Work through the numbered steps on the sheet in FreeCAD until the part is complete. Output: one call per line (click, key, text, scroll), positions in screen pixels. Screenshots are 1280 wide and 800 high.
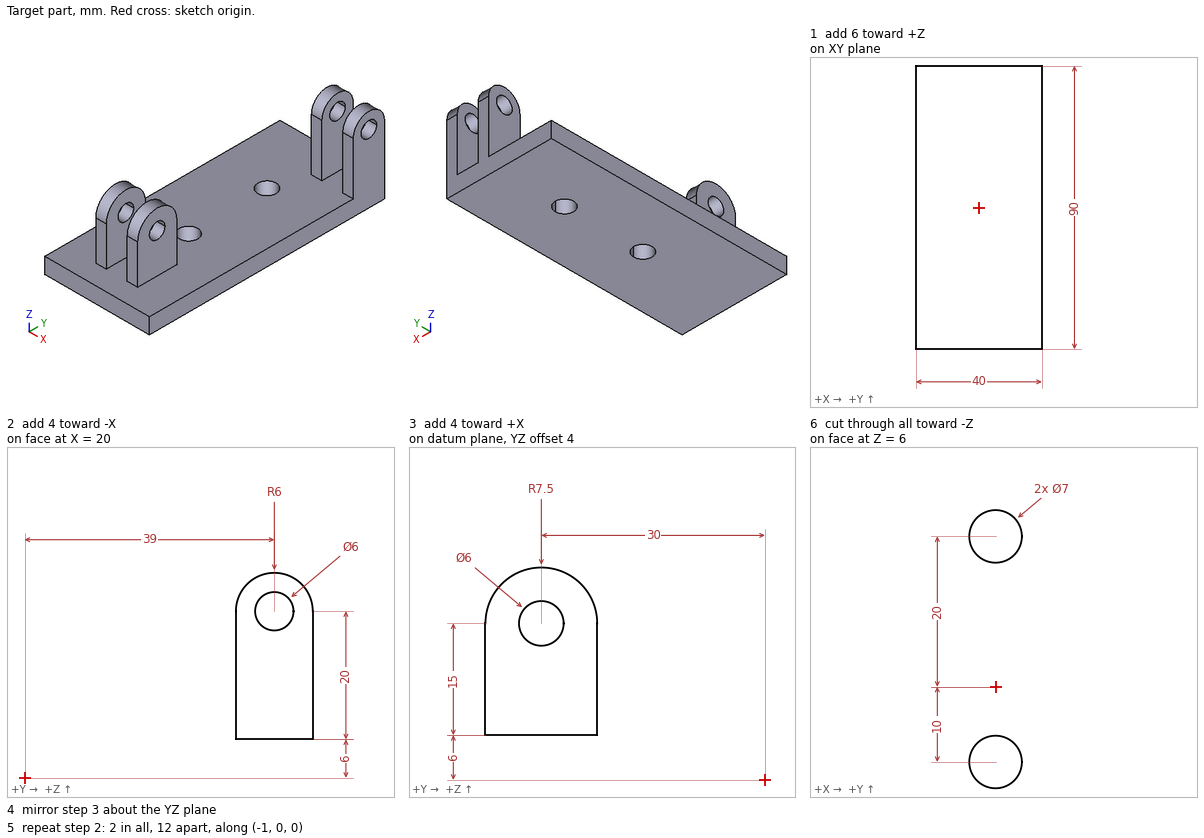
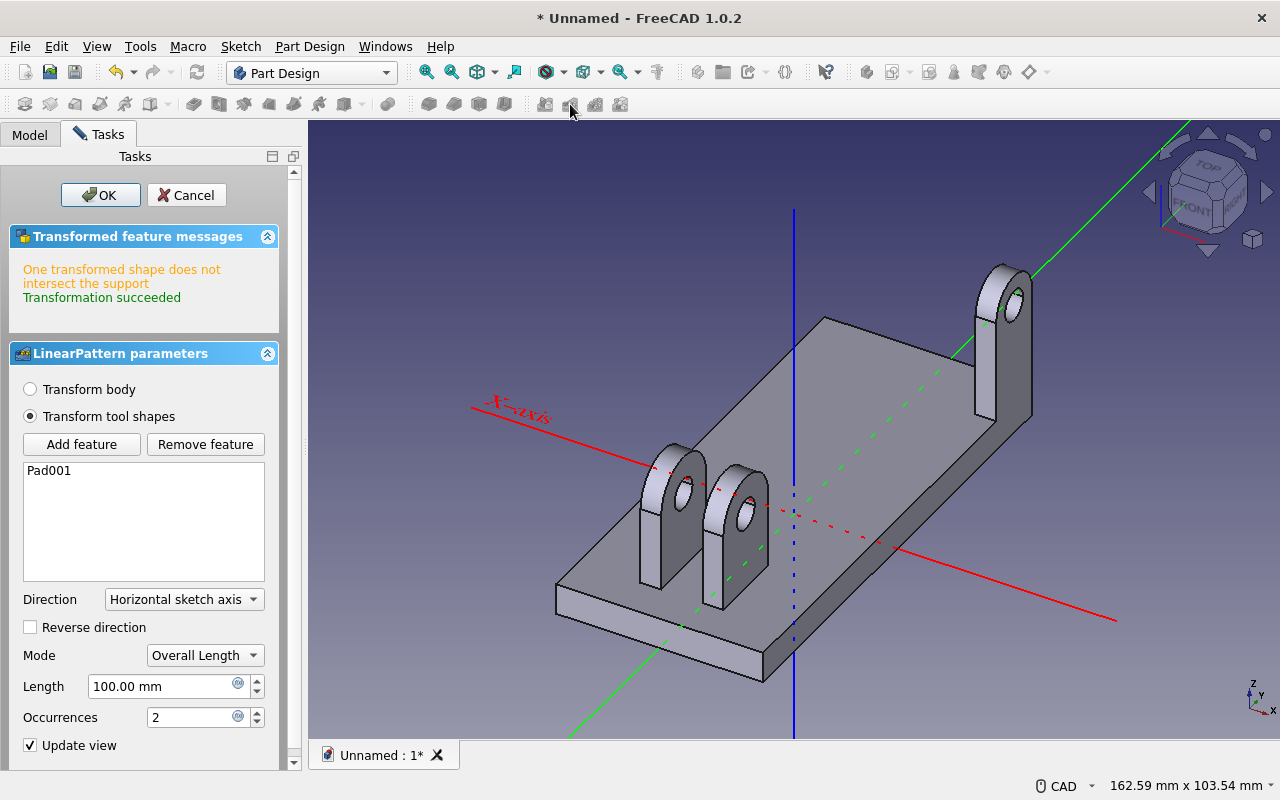
click(185, 600)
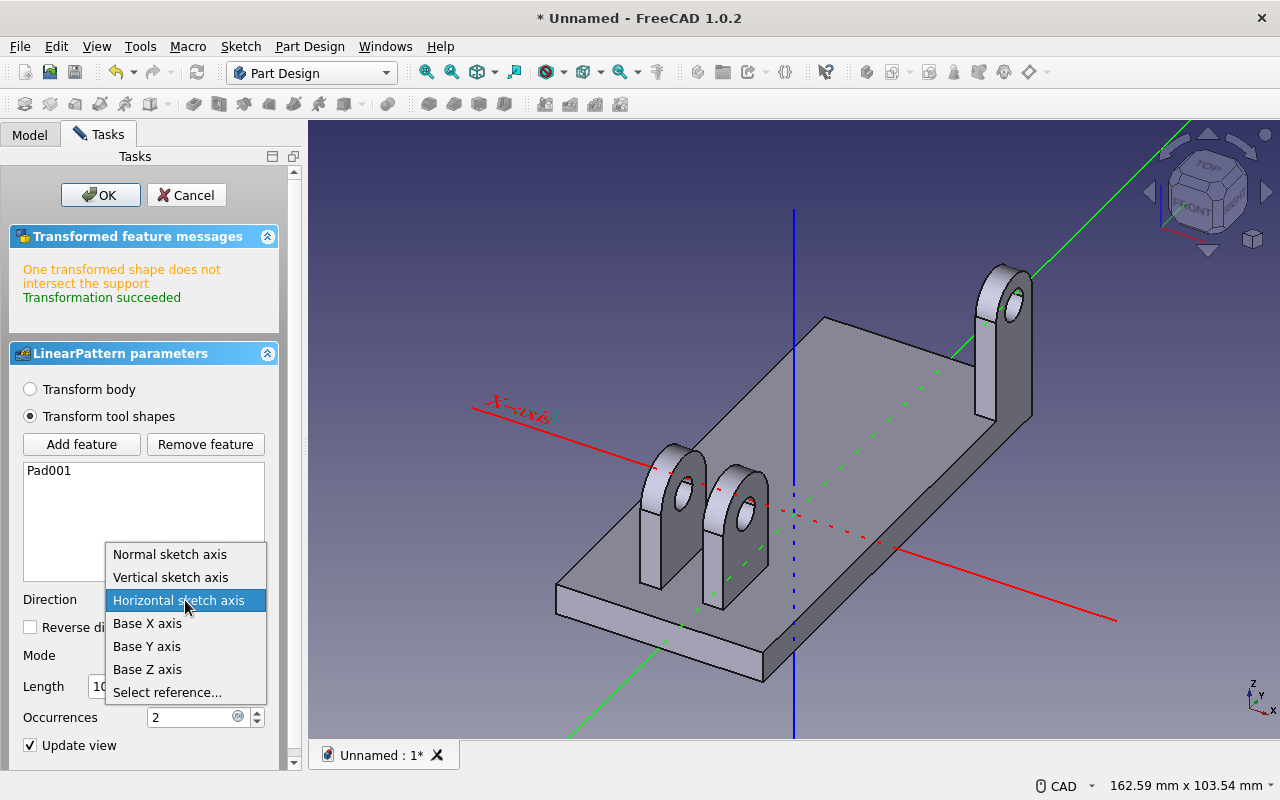
click(184, 624)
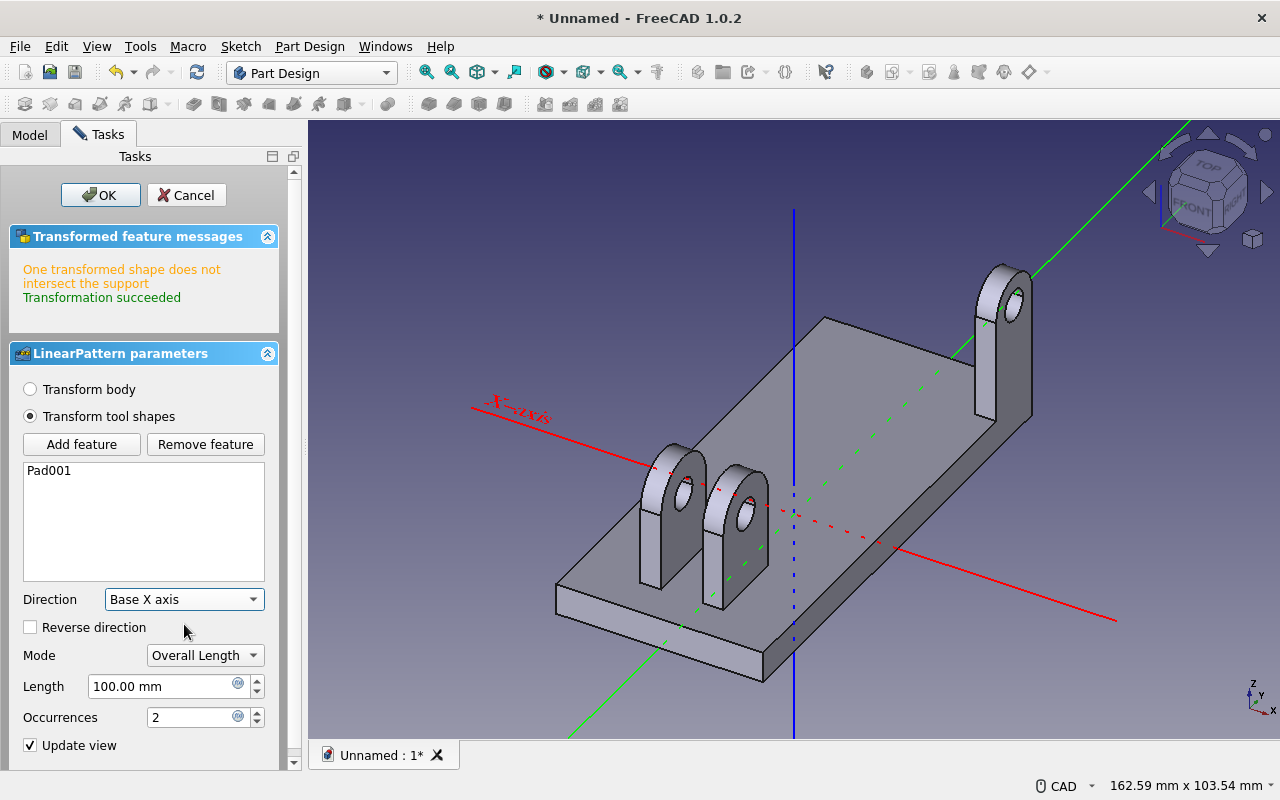
click(206, 656)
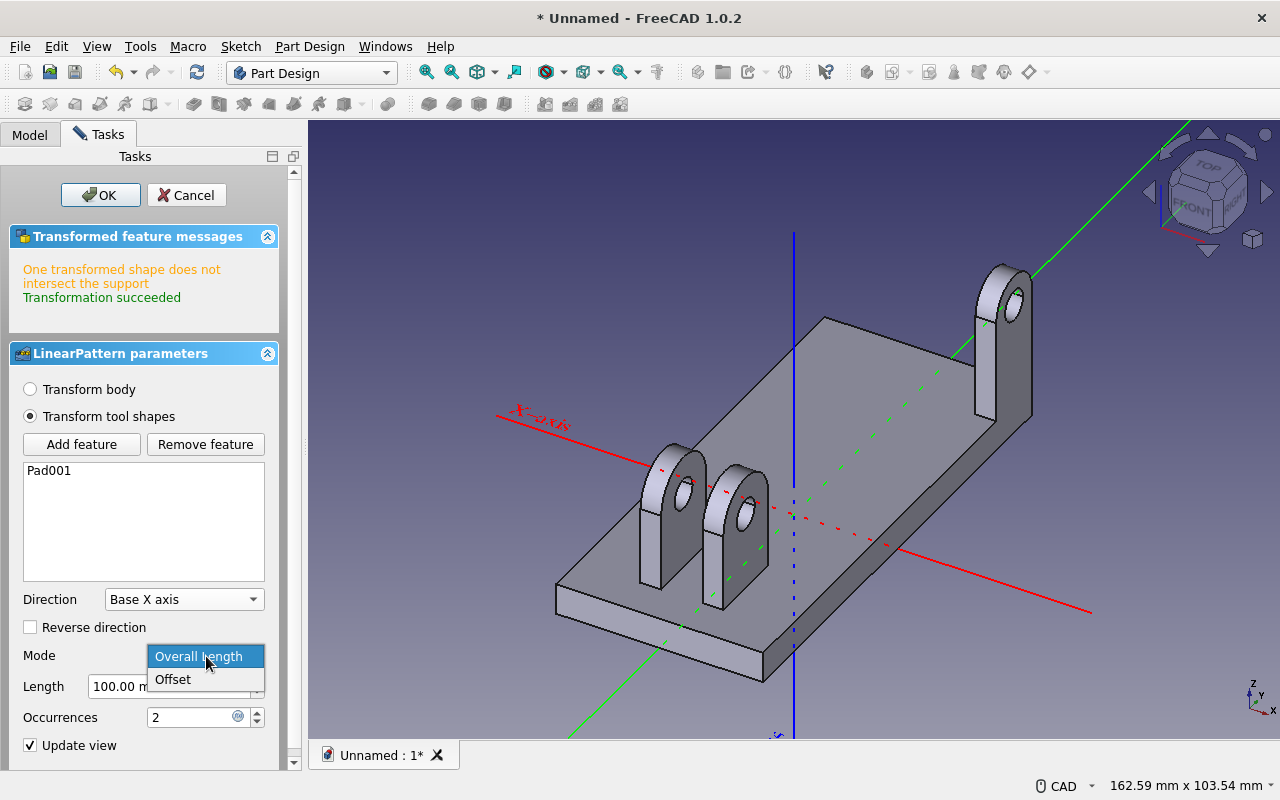
click(204, 680)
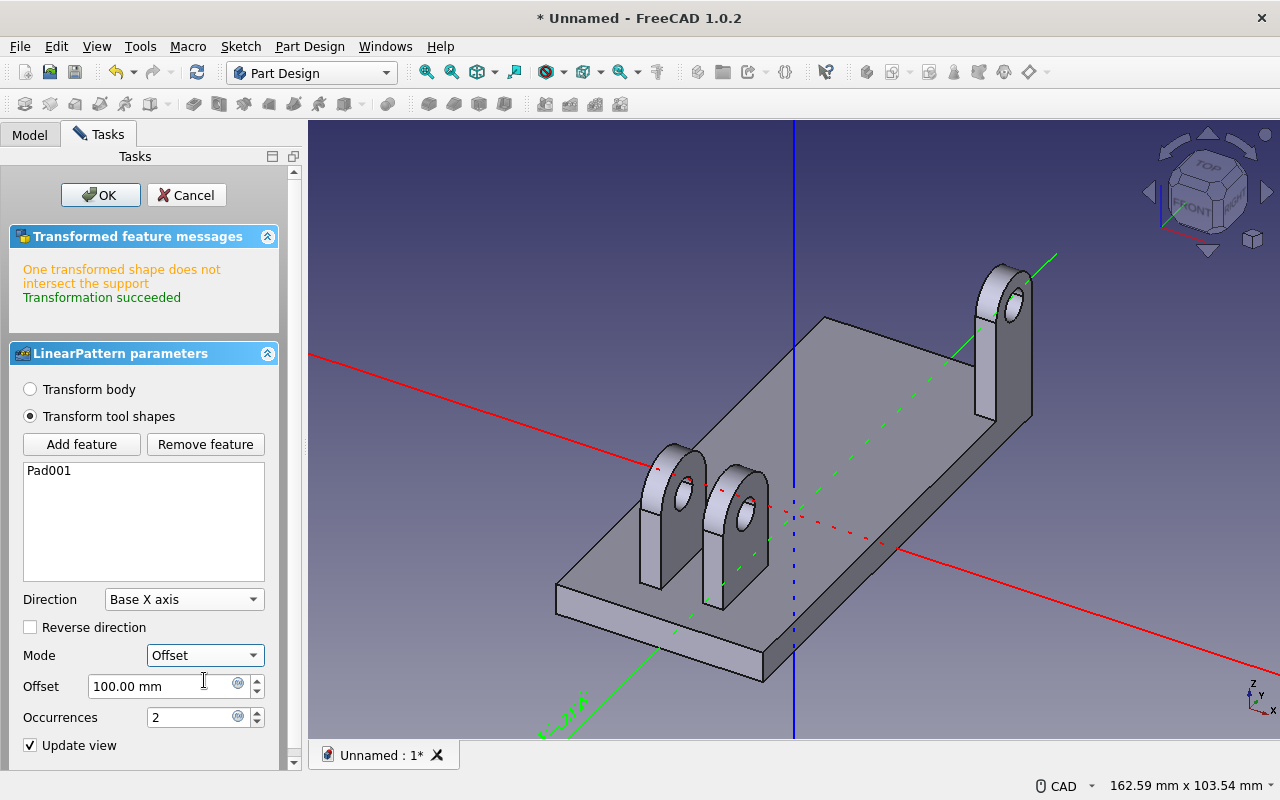
triple_click(170, 686)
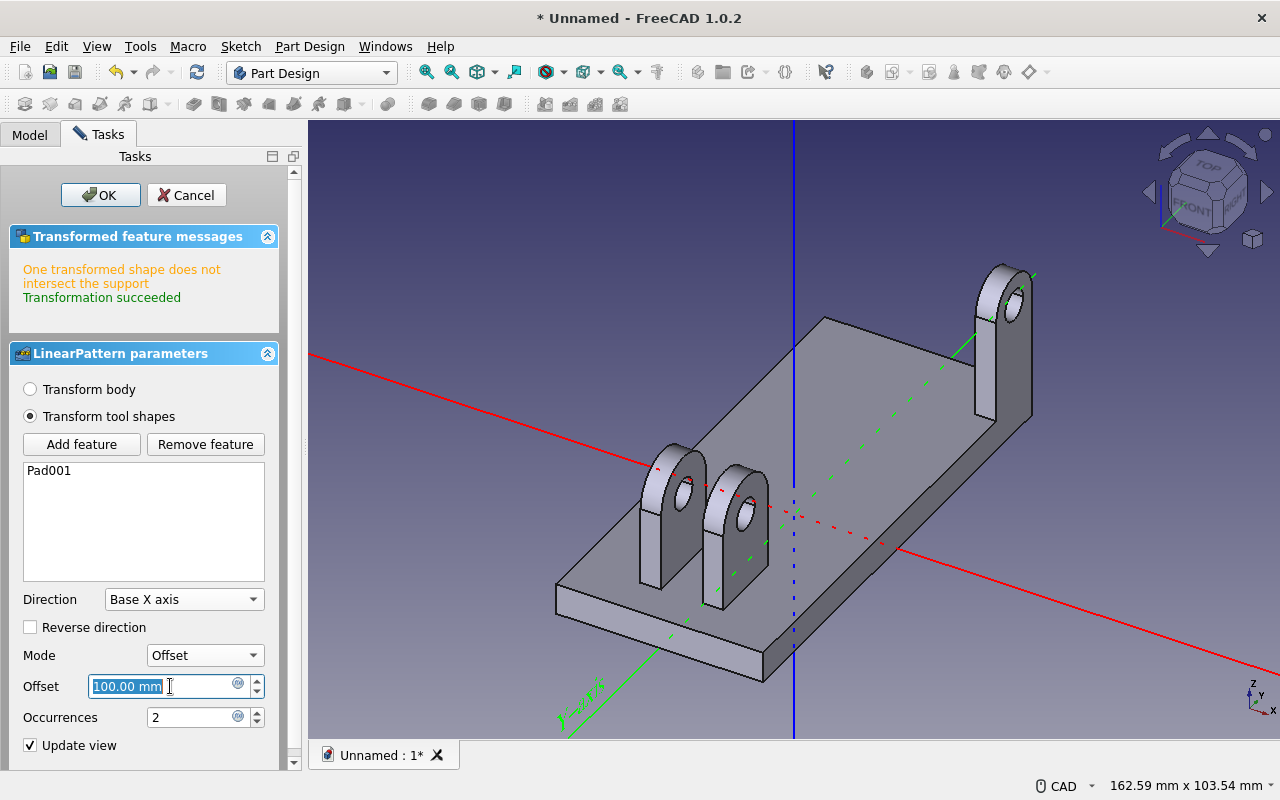
text(12)
key(Tab)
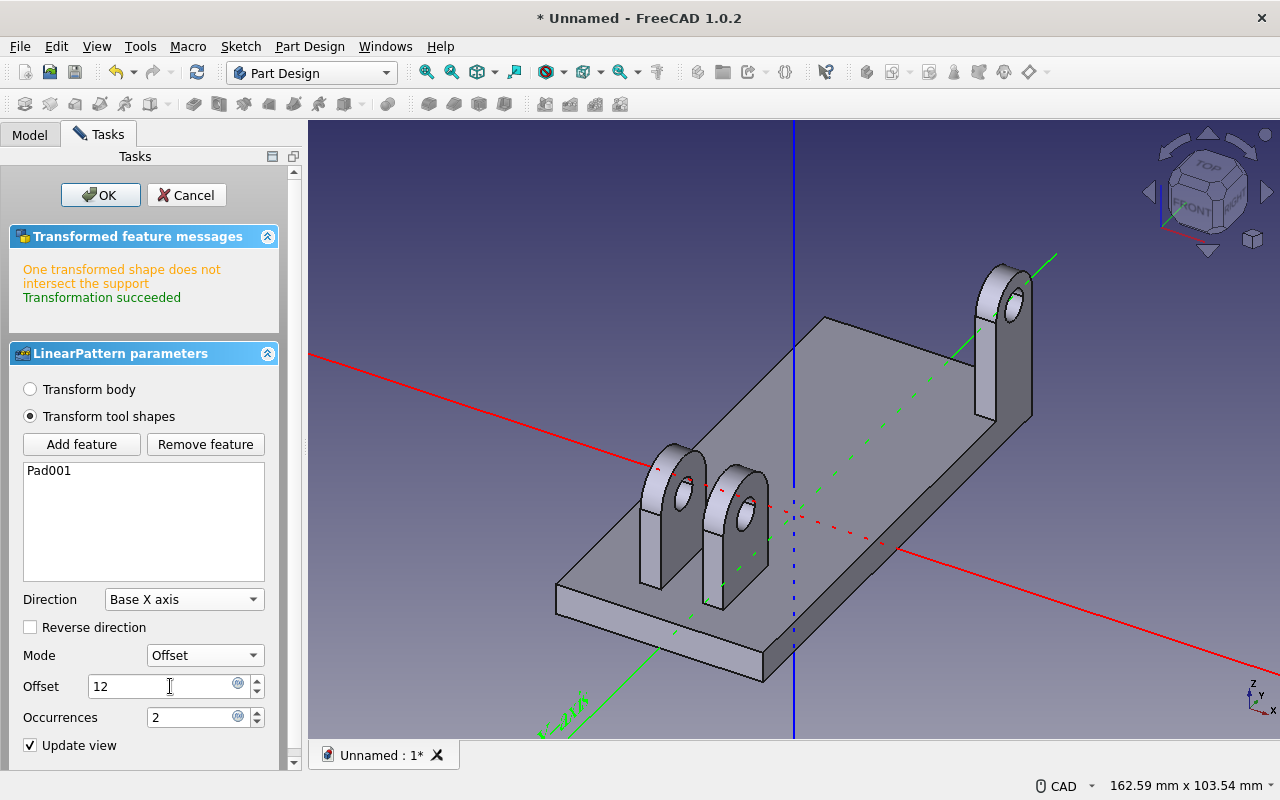
triple_click(199, 718)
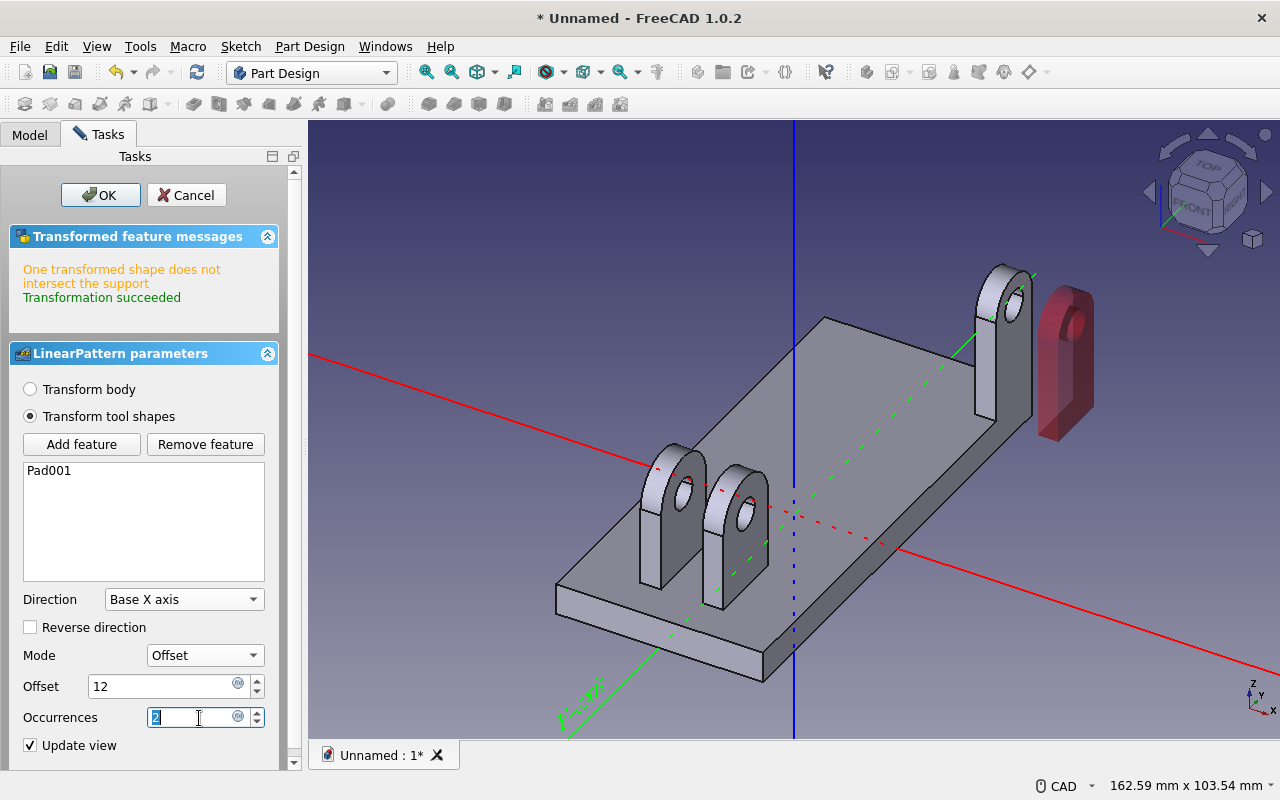
text(2)
key(Tab)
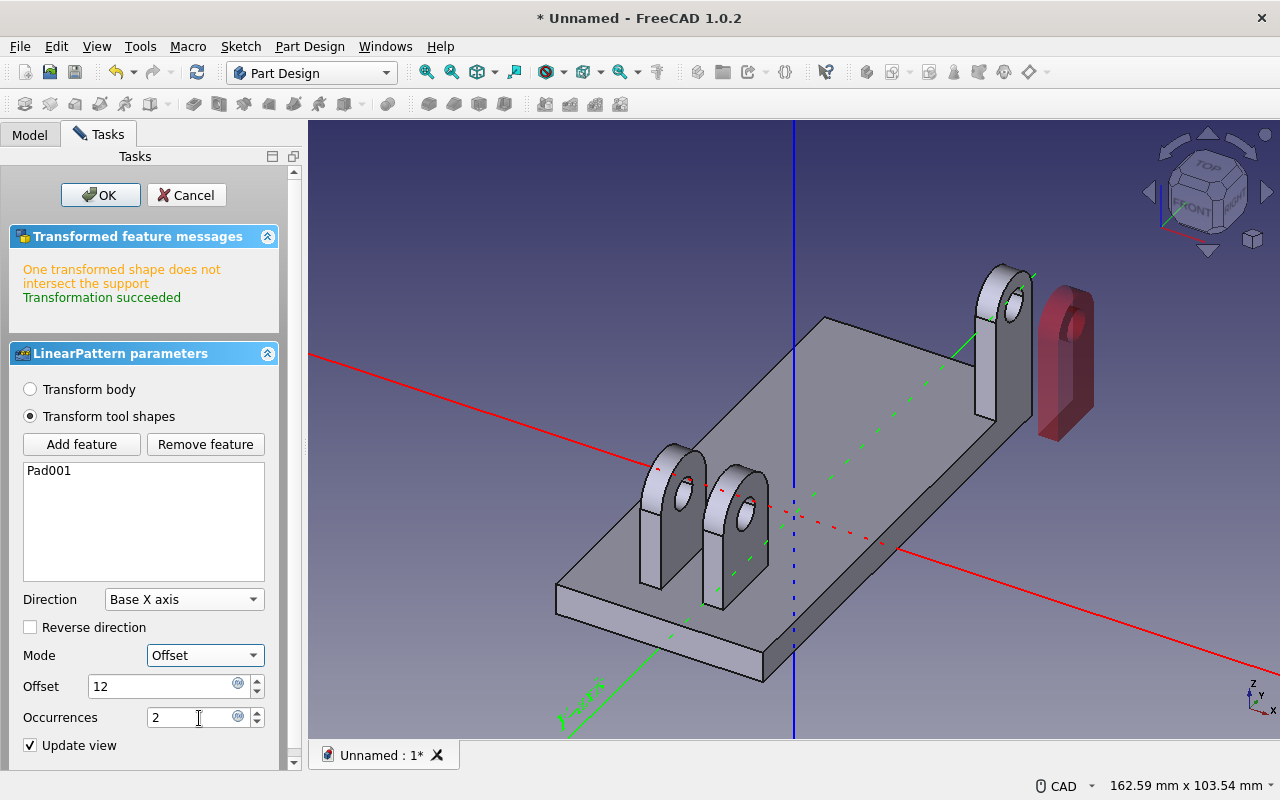
click(31, 627)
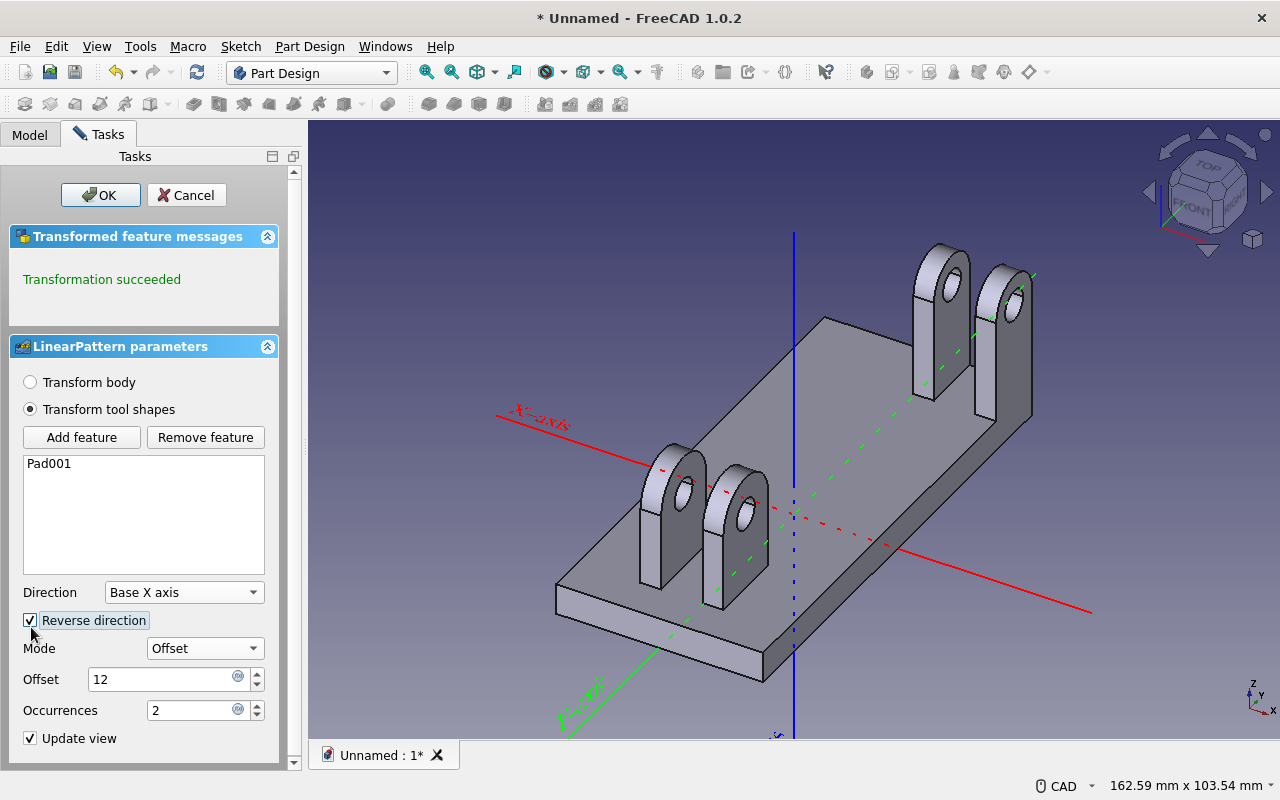
click(101, 195)